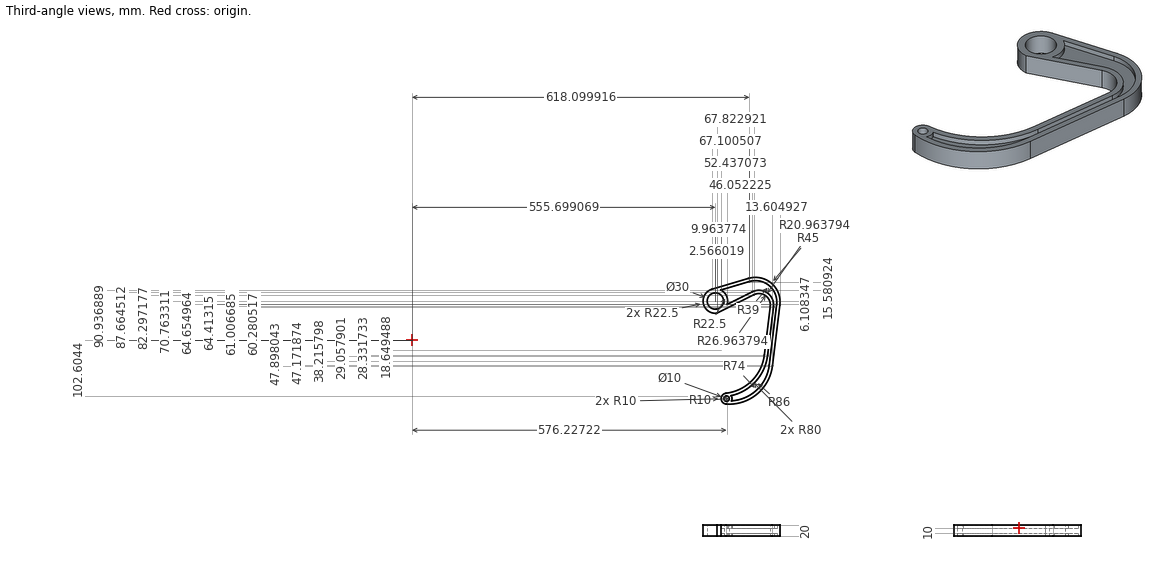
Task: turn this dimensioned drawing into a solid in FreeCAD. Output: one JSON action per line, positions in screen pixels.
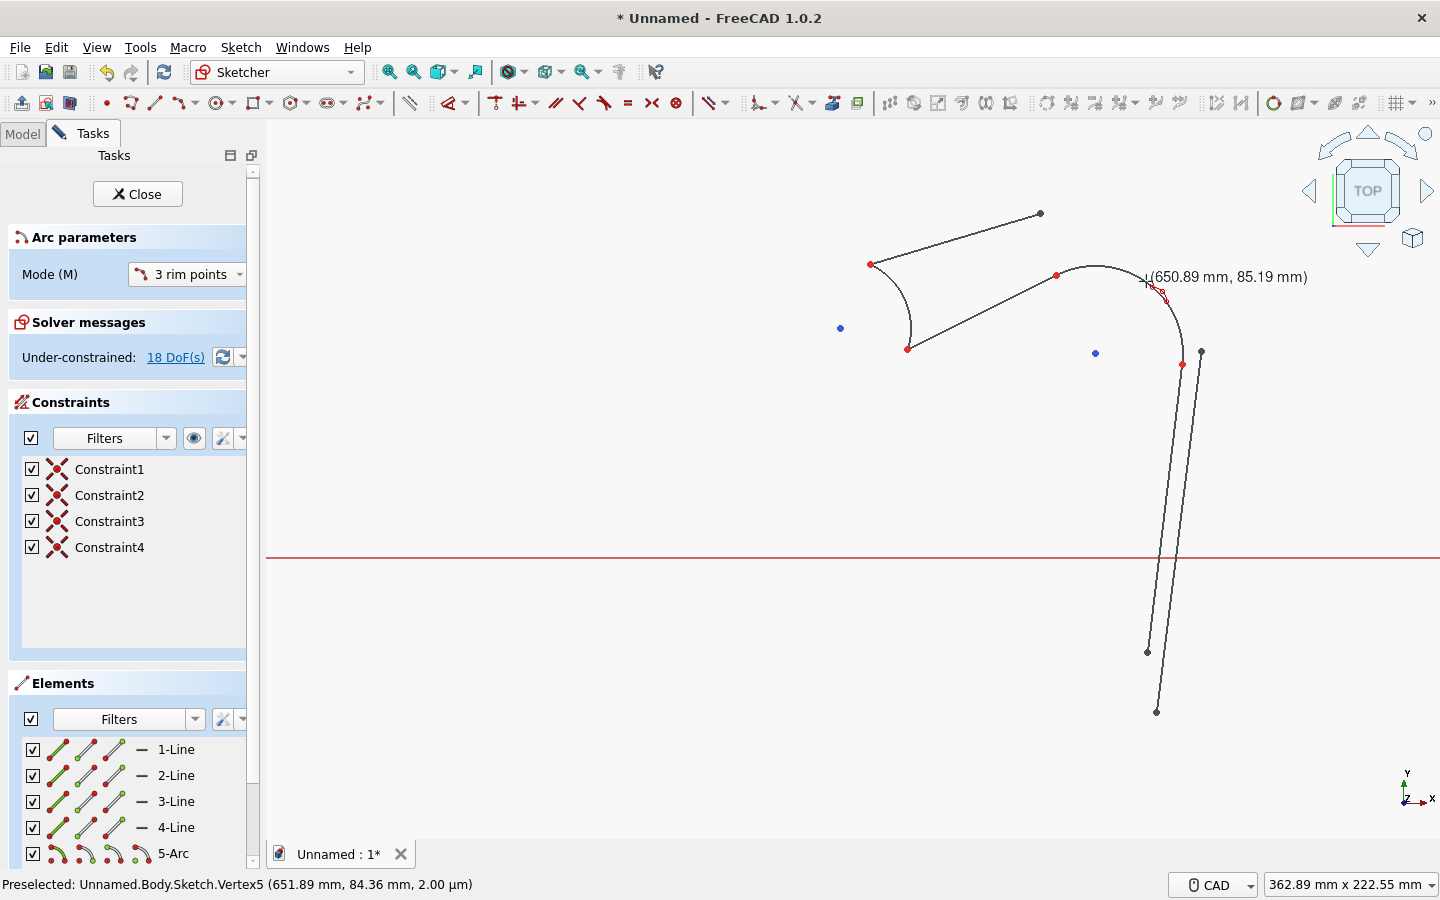
{"action": "left_click", "coordinate": [1148, 652]}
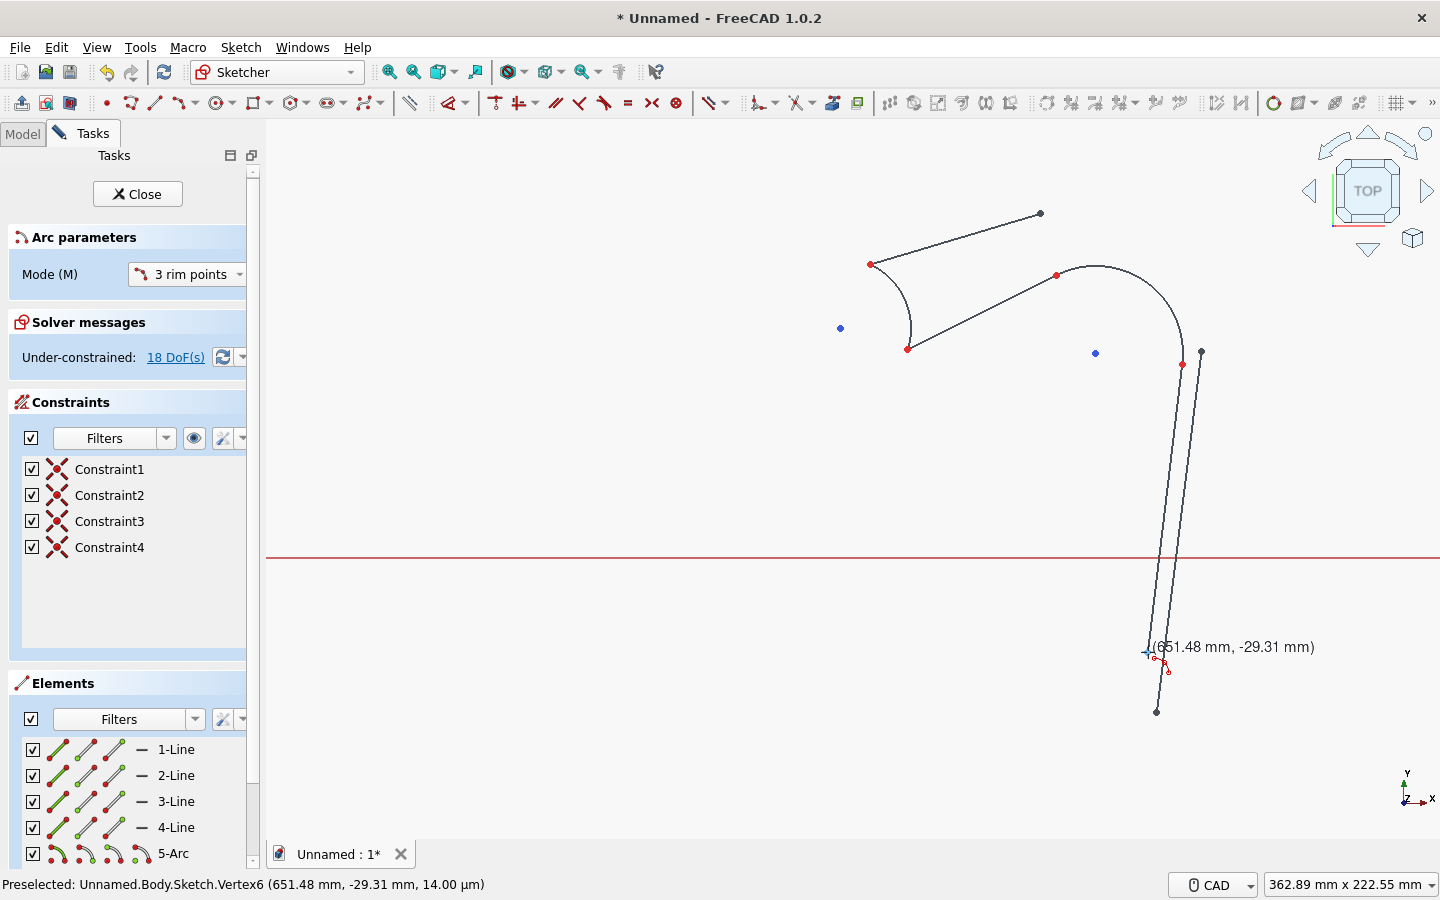
{"action": "scroll", "coordinate": [294, 301], "scroll_direction": "down", "scroll_amount": 2}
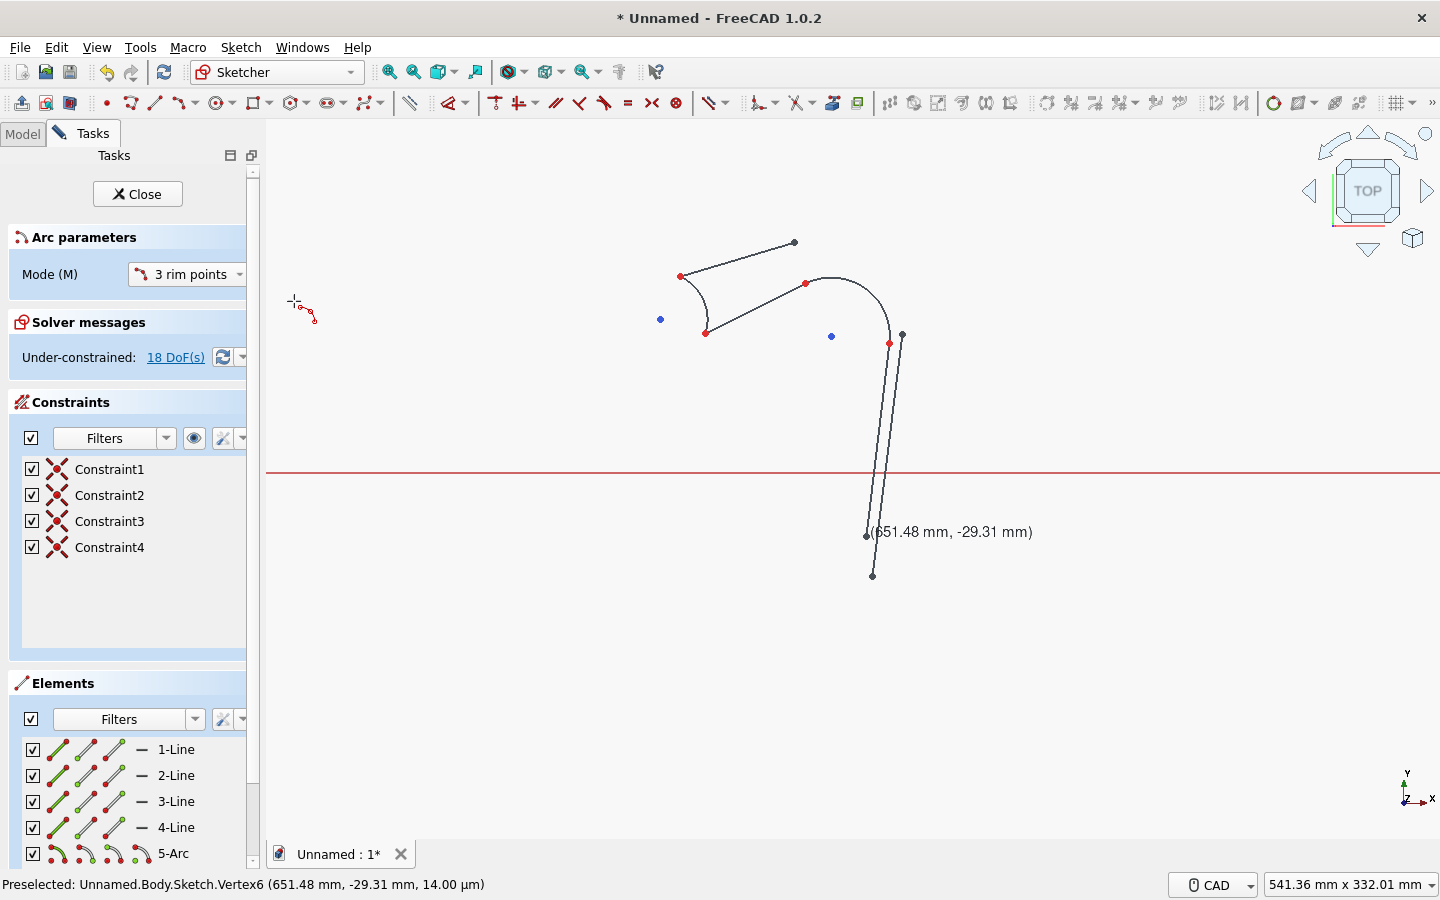
{"action": "left_click", "coordinate": [721, 696]}
{"action": "left_click", "coordinate": [819, 639]}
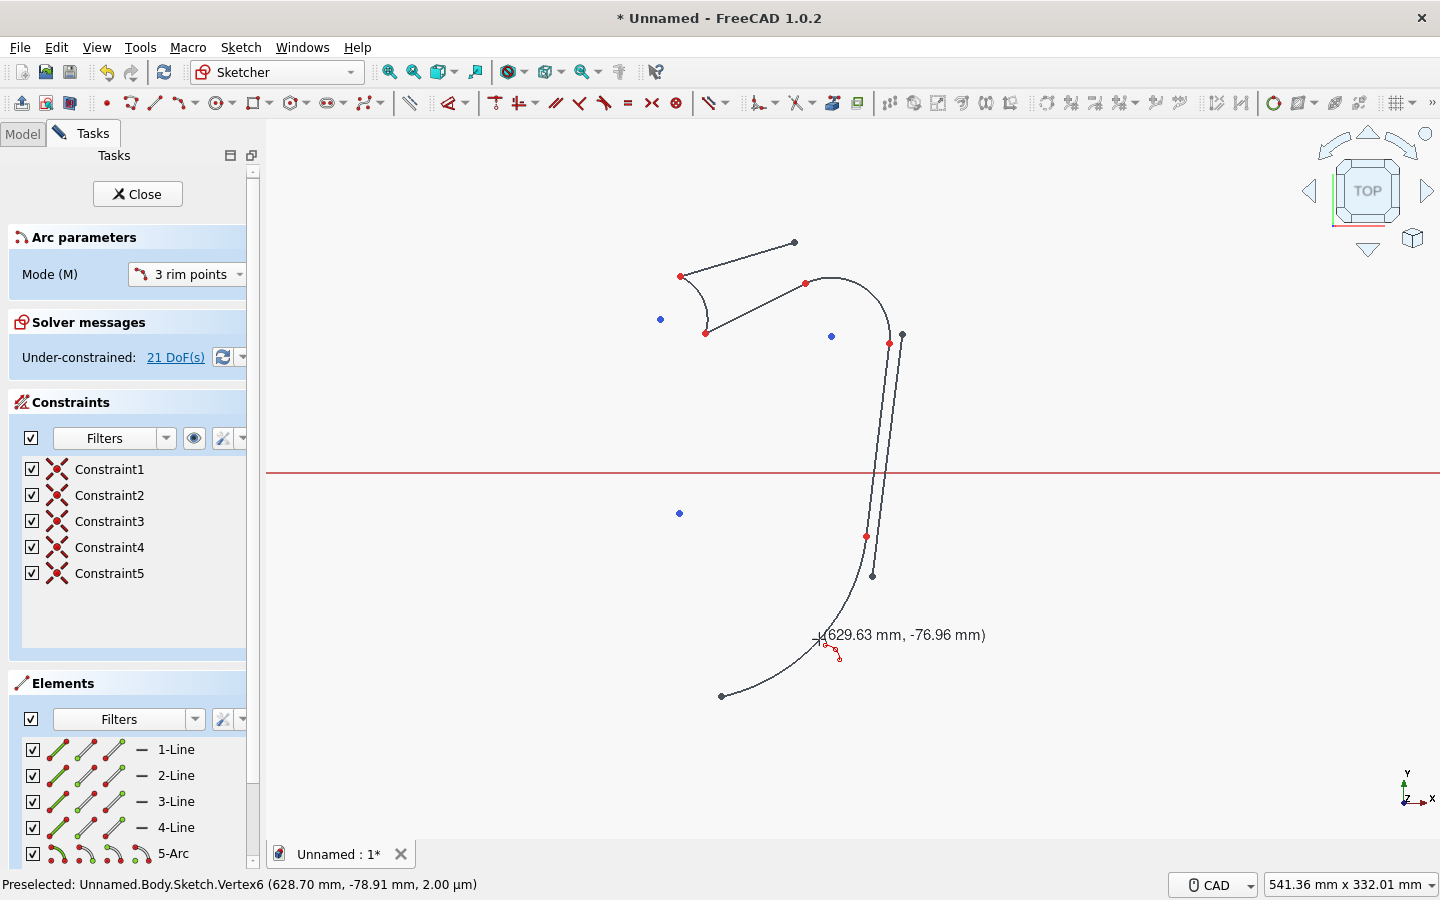
{"action": "left_click", "coordinate": [721, 697]}
{"action": "left_click", "coordinate": [723, 716]}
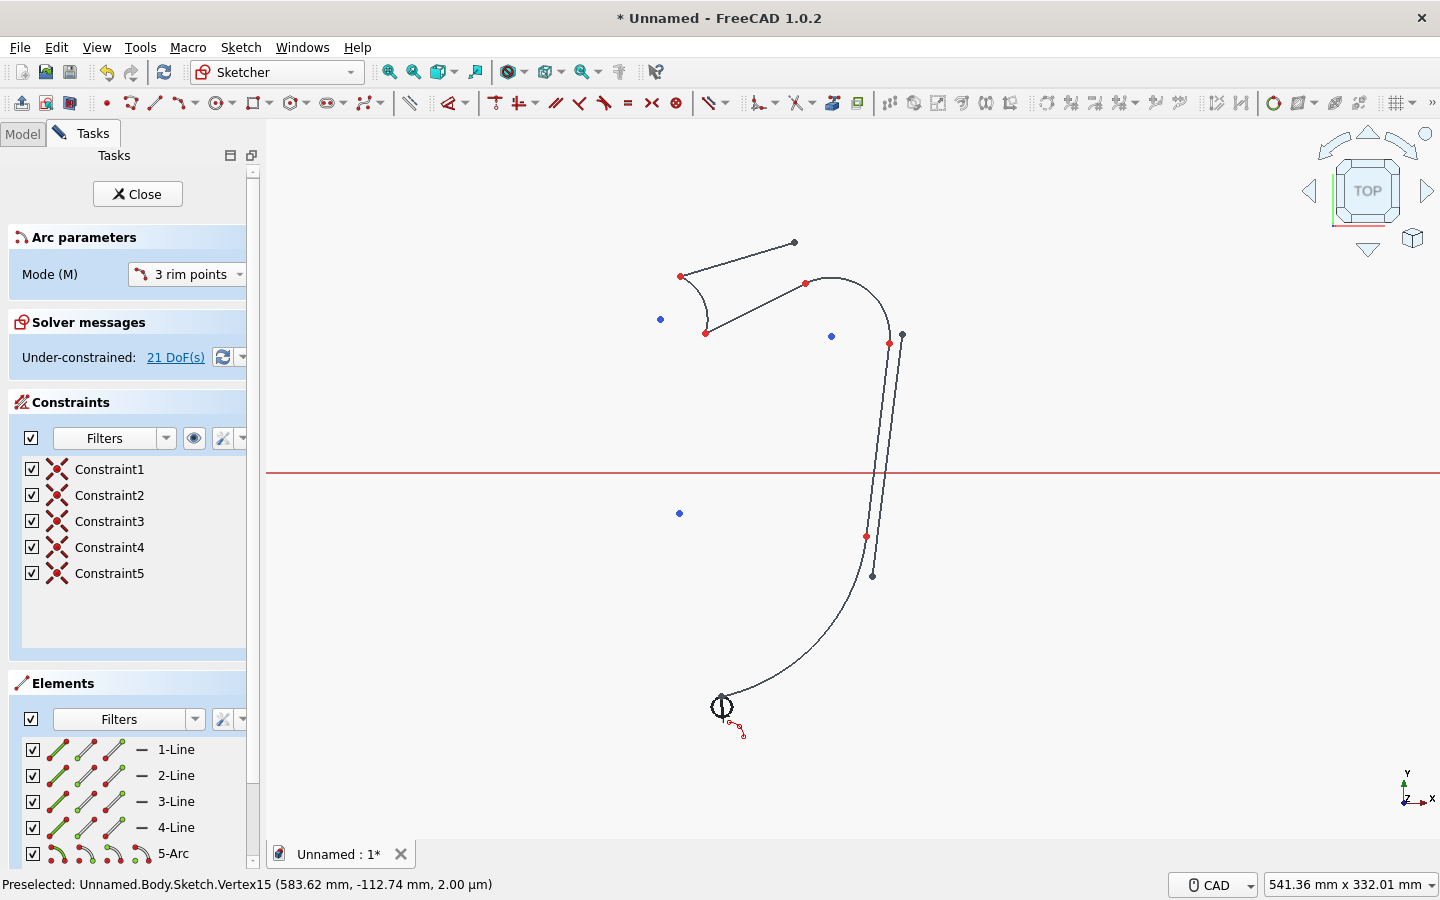
{"action": "scroll", "coordinate": [725, 706], "scroll_direction": "up", "scroll_amount": 10}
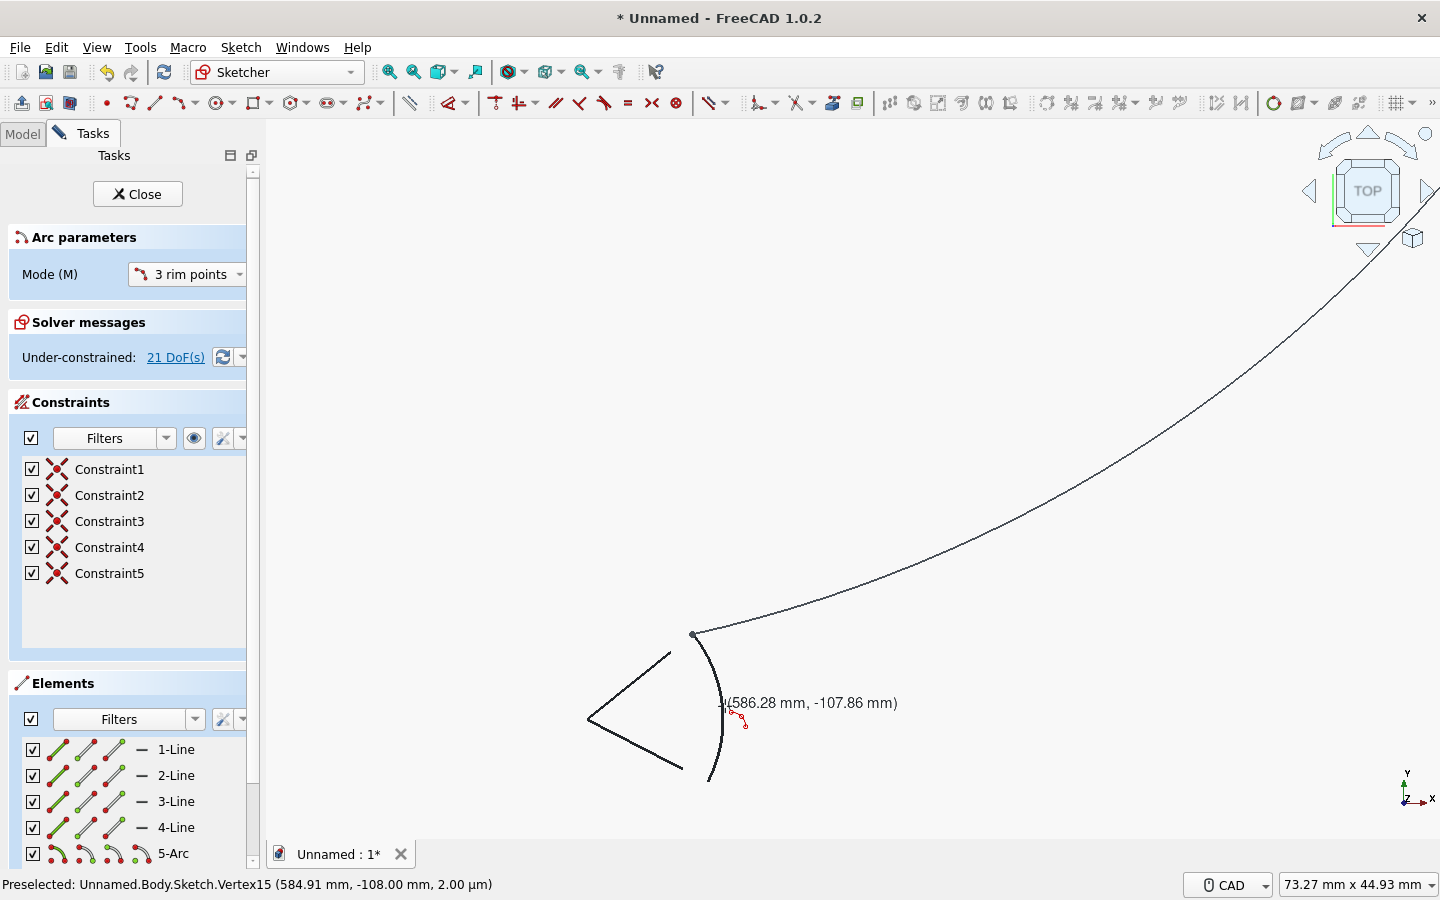
{"action": "left_click", "coordinate": [721, 698]}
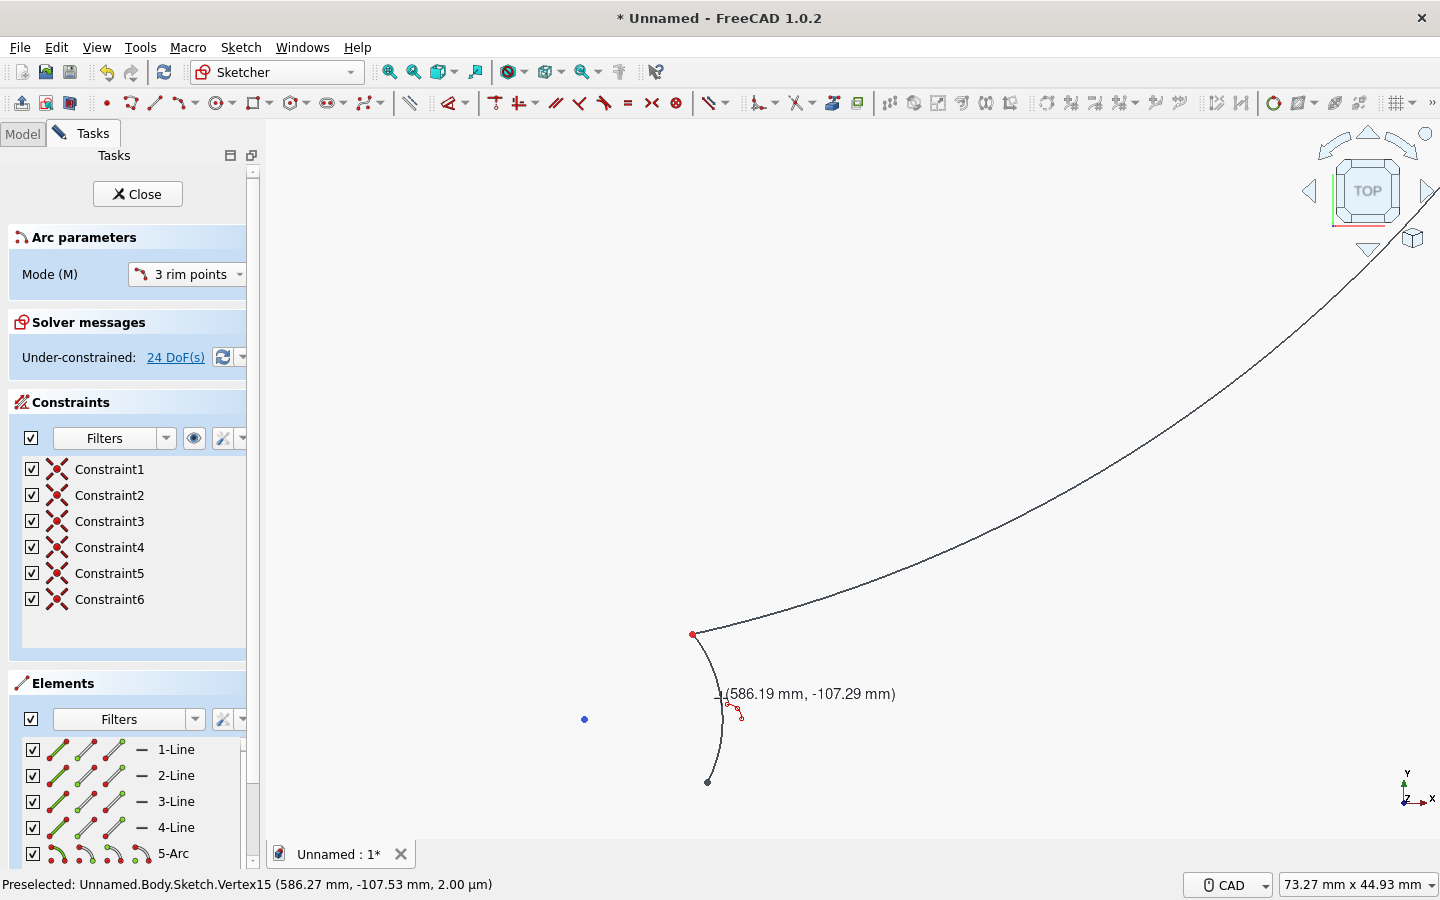
{"action": "scroll", "coordinate": [718, 707], "scroll_direction": "down", "scroll_amount": 10}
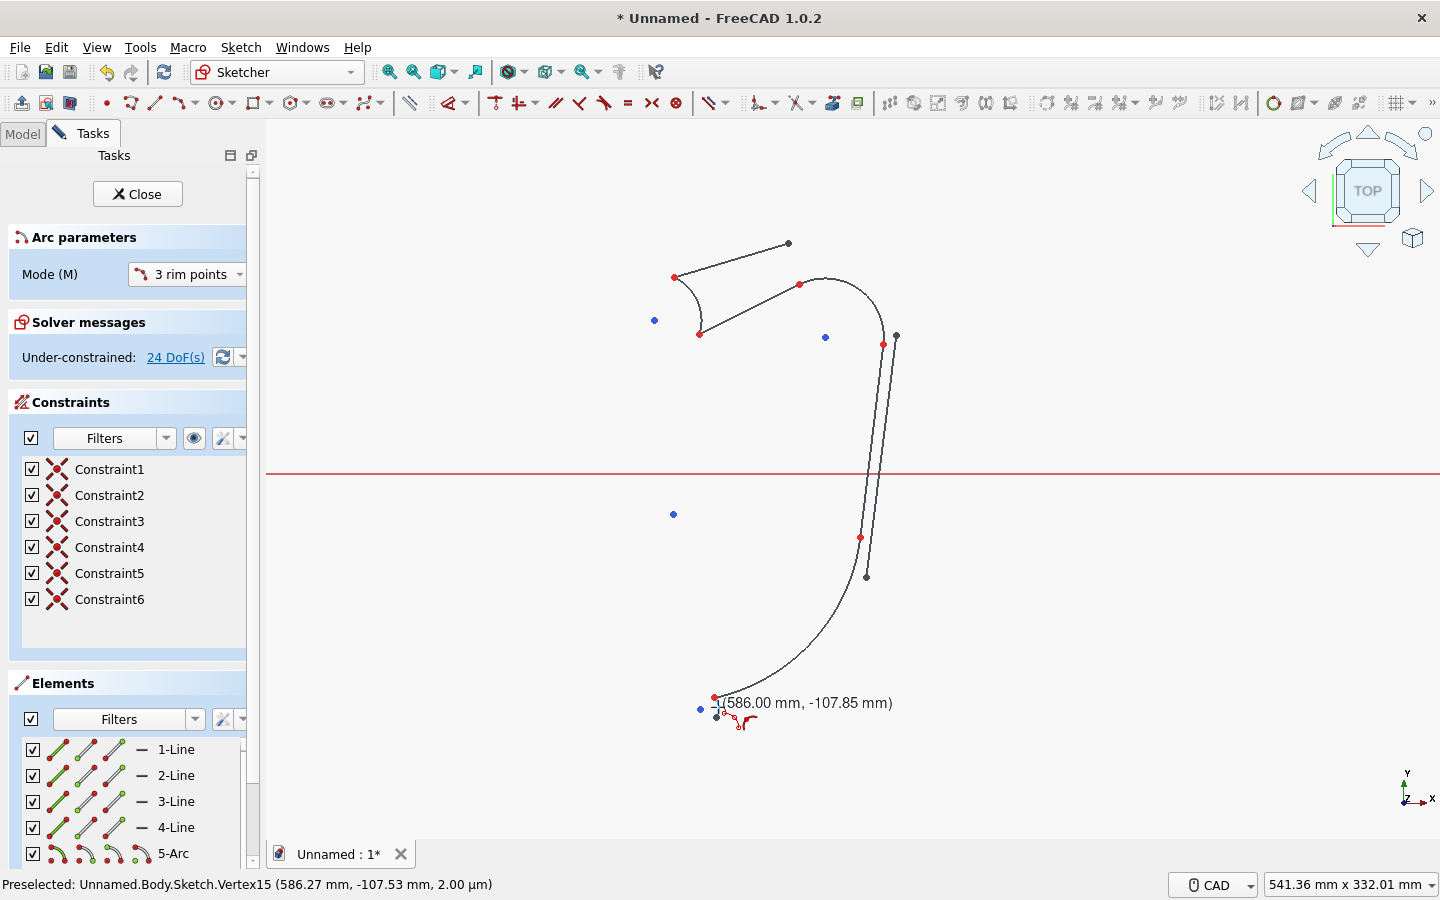
{"action": "left_click", "coordinate": [717, 718]}
{"action": "left_click", "coordinate": [866, 578]}
{"action": "left_click", "coordinate": [817, 674]}